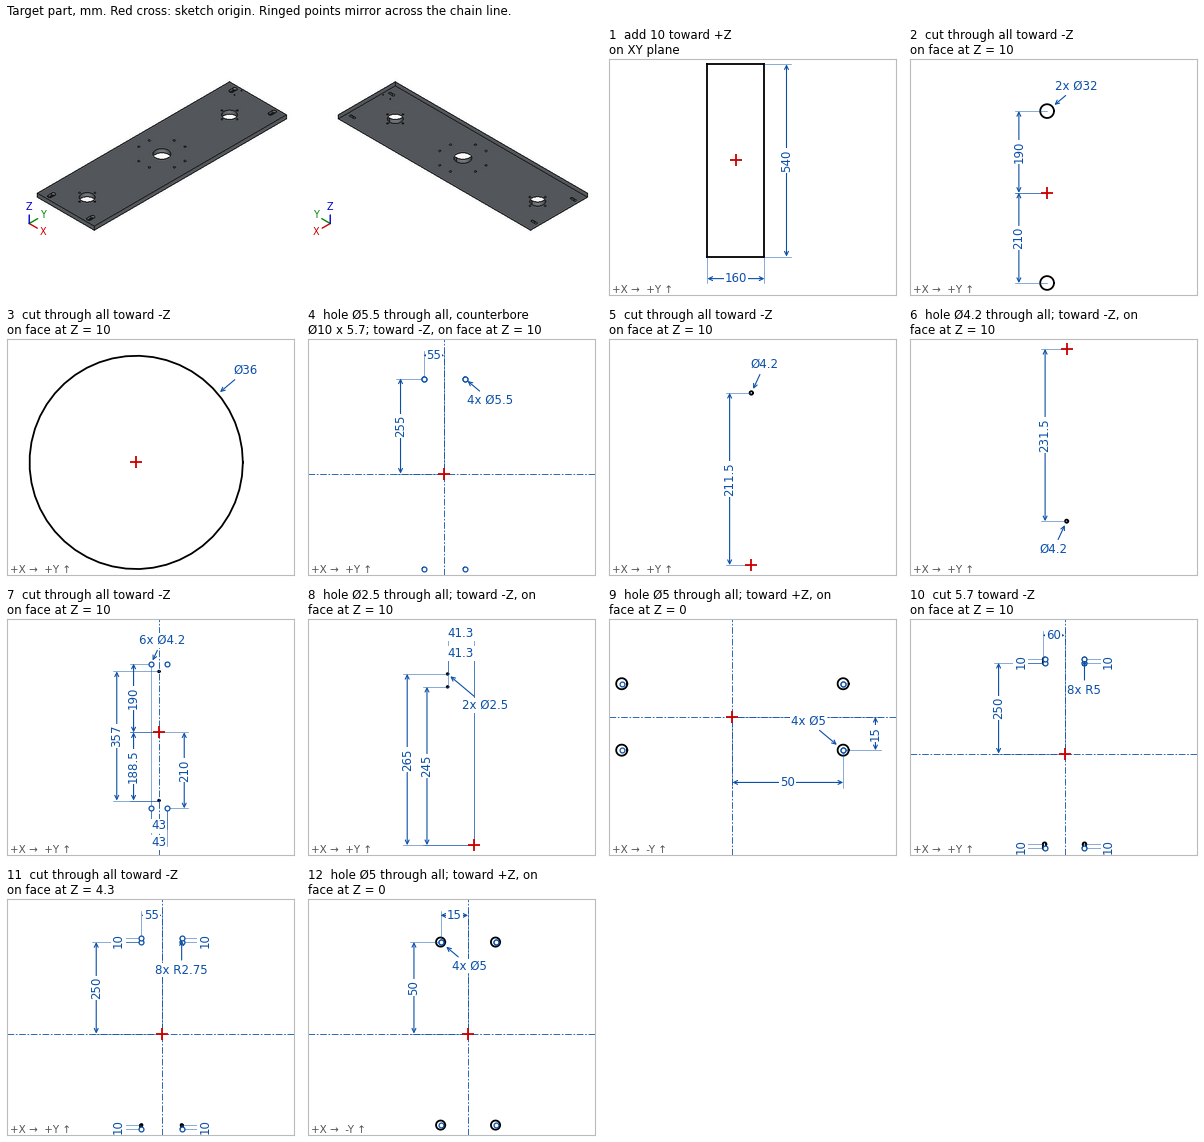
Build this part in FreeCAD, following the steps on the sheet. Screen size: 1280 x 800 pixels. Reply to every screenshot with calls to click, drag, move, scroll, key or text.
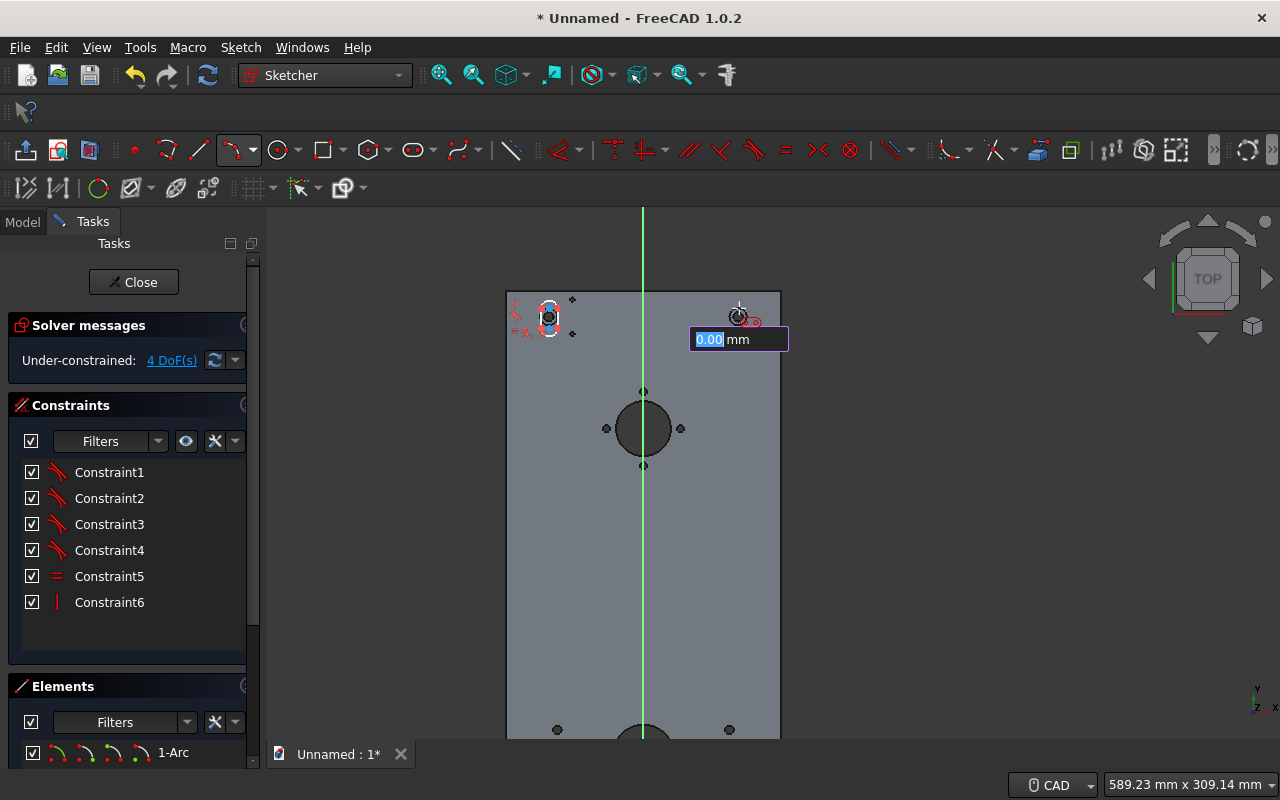
scroll(747, 317, up, 4)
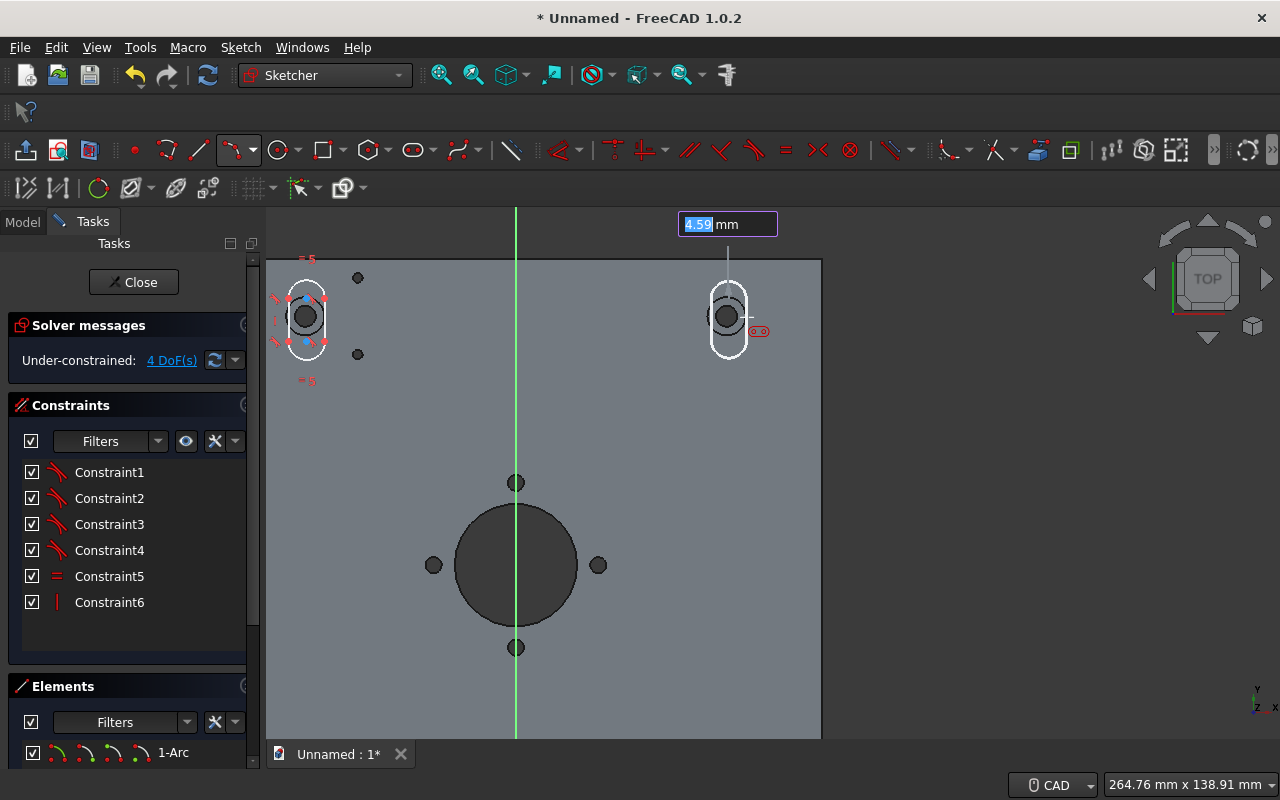
click(746, 316)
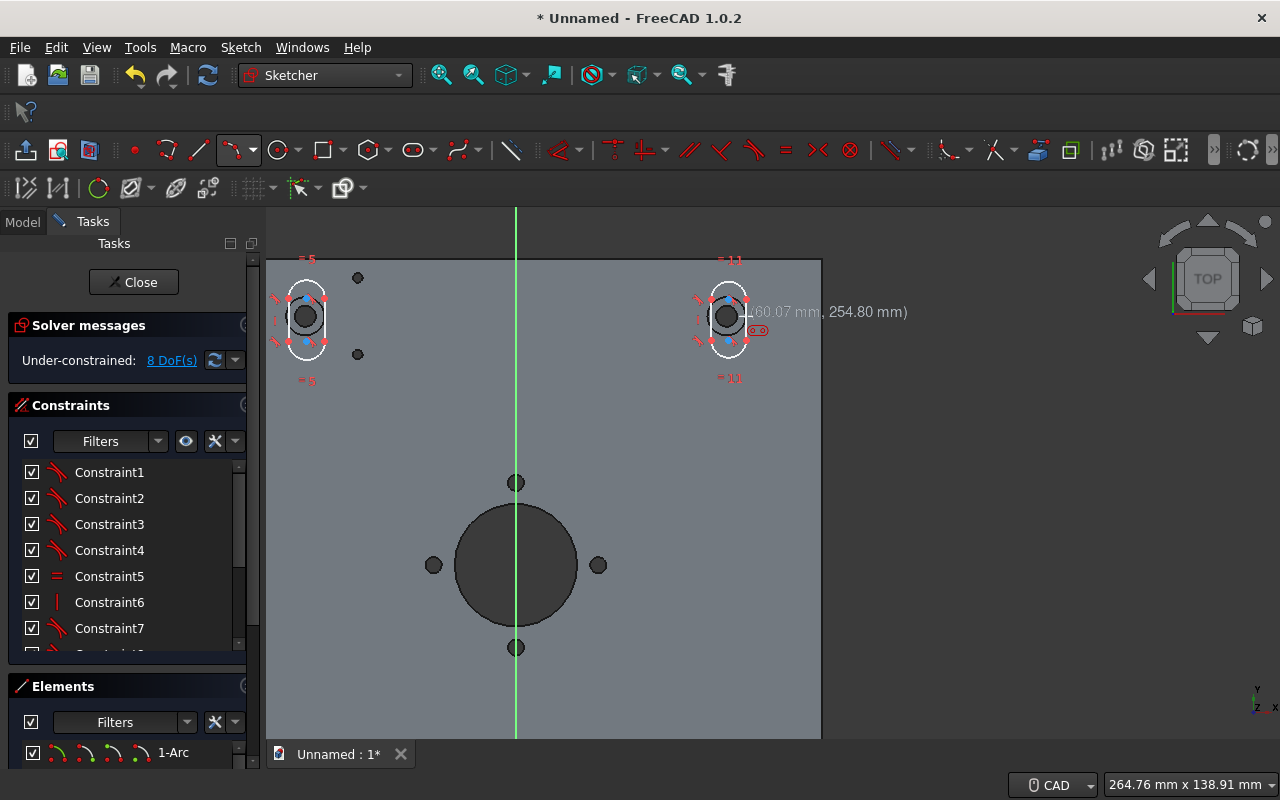
scroll(742, 311, down, 9)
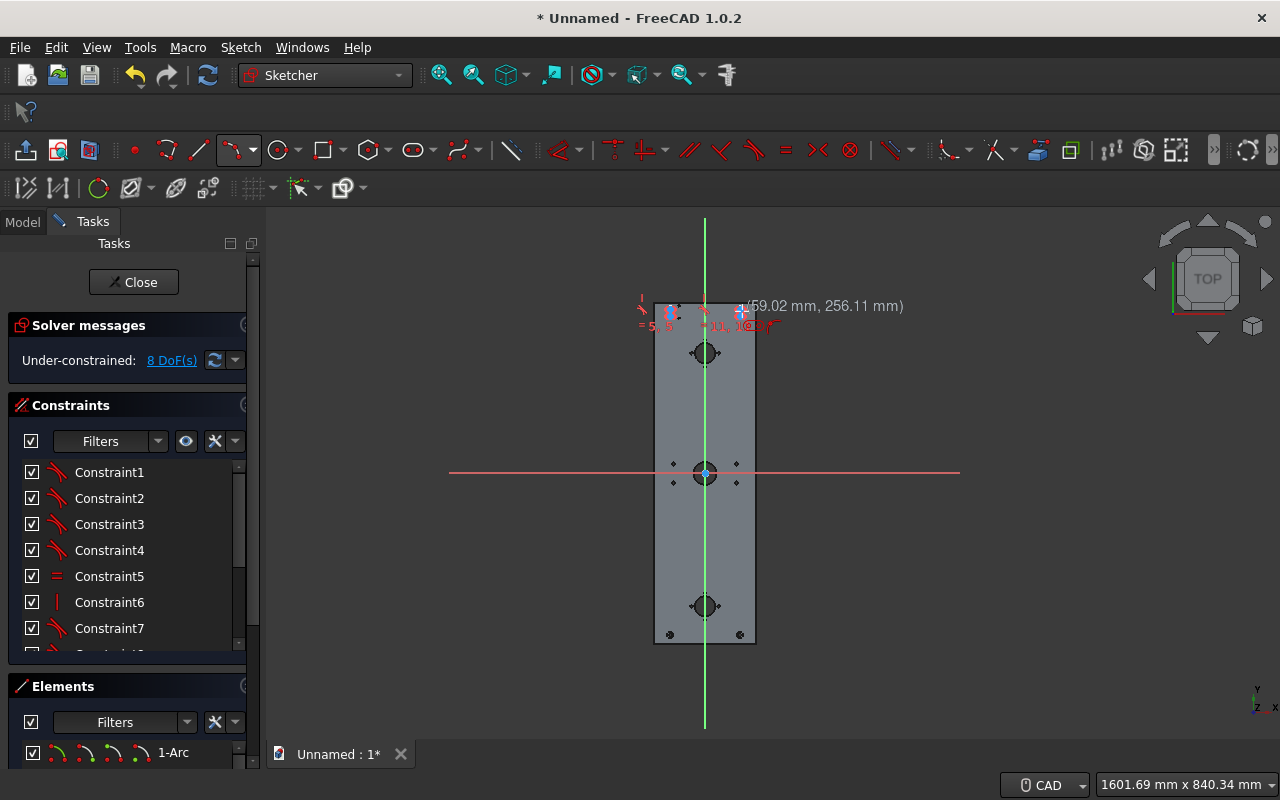
scroll(670, 638, up, 10)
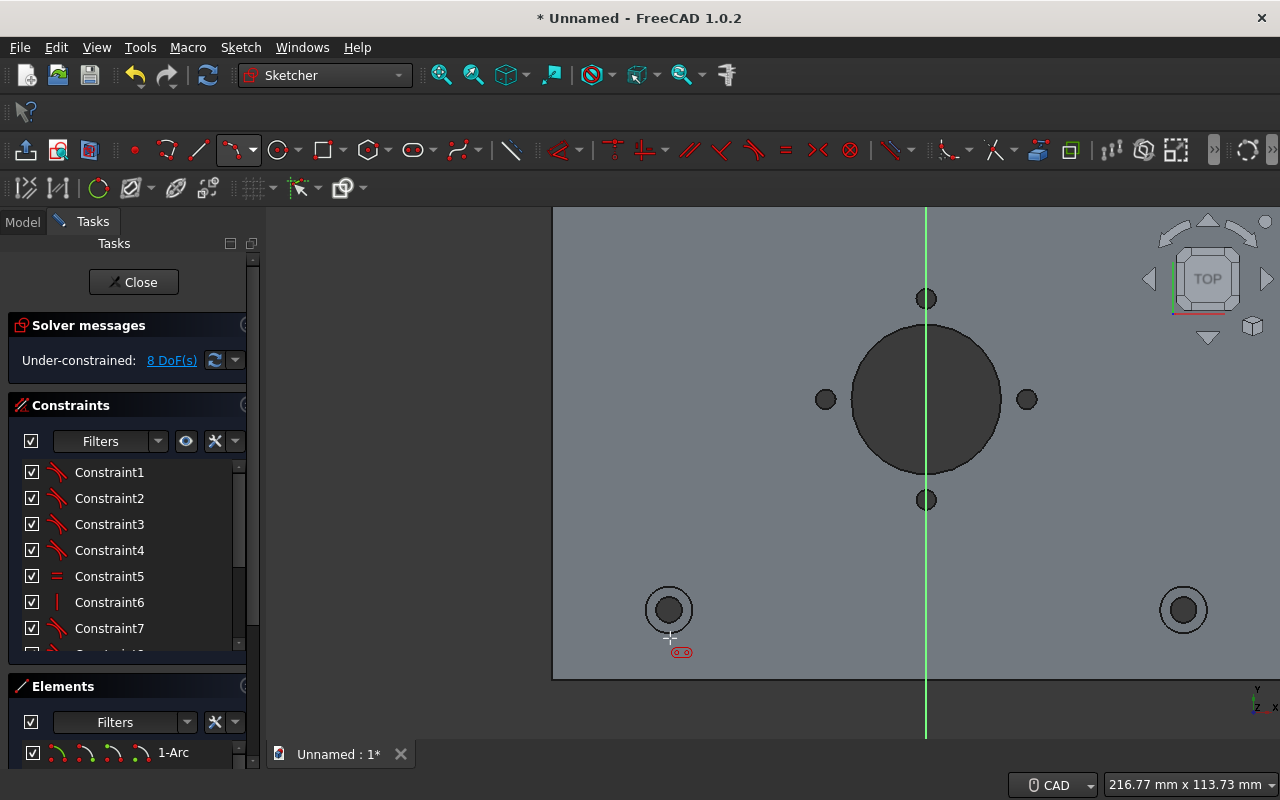
scroll(670, 638, down, 10)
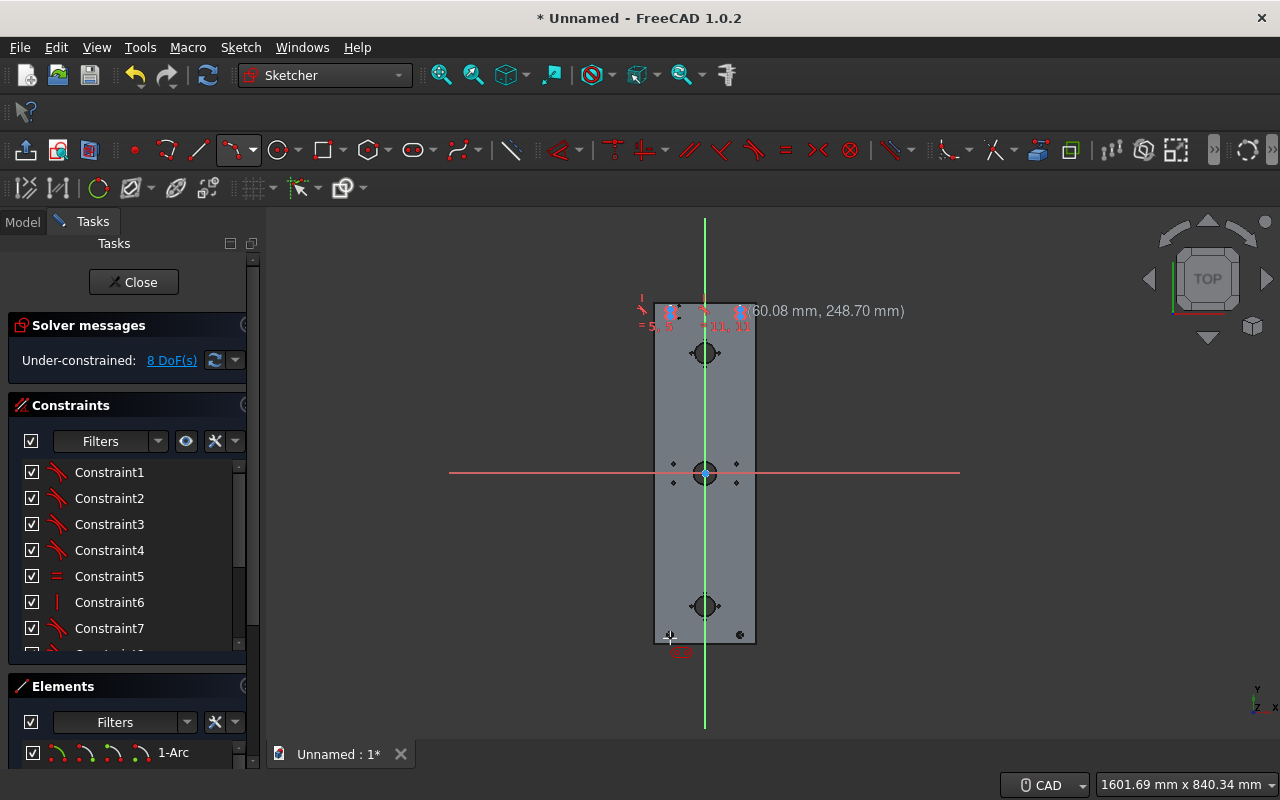
click(670, 638)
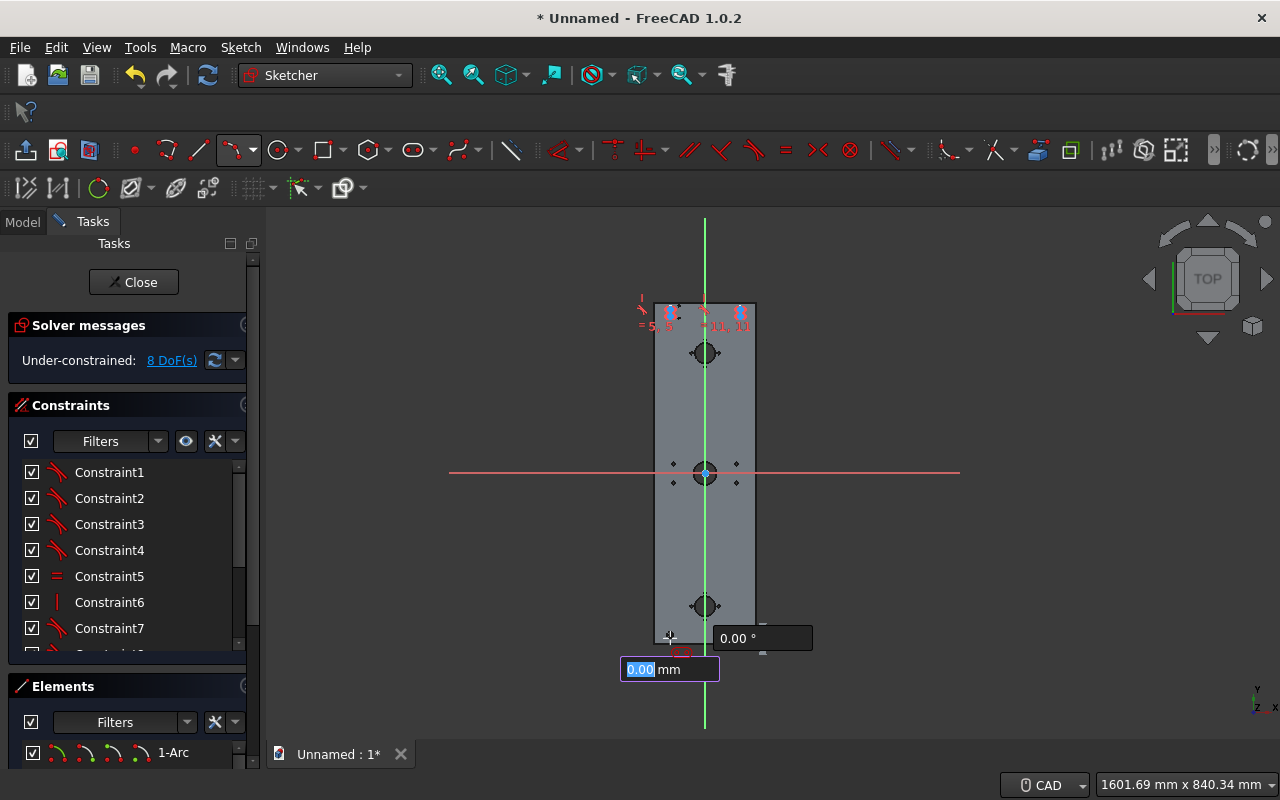
scroll(670, 632, up, 5)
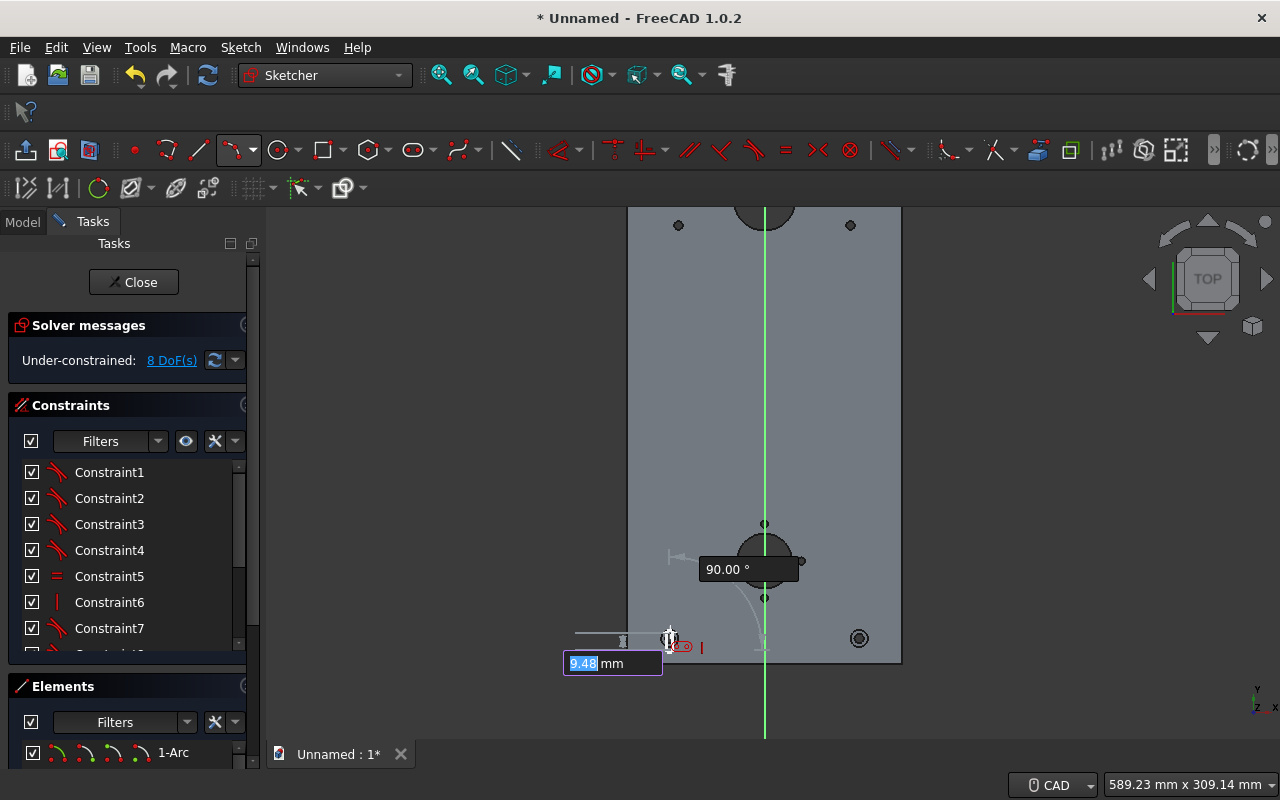
click(669, 630)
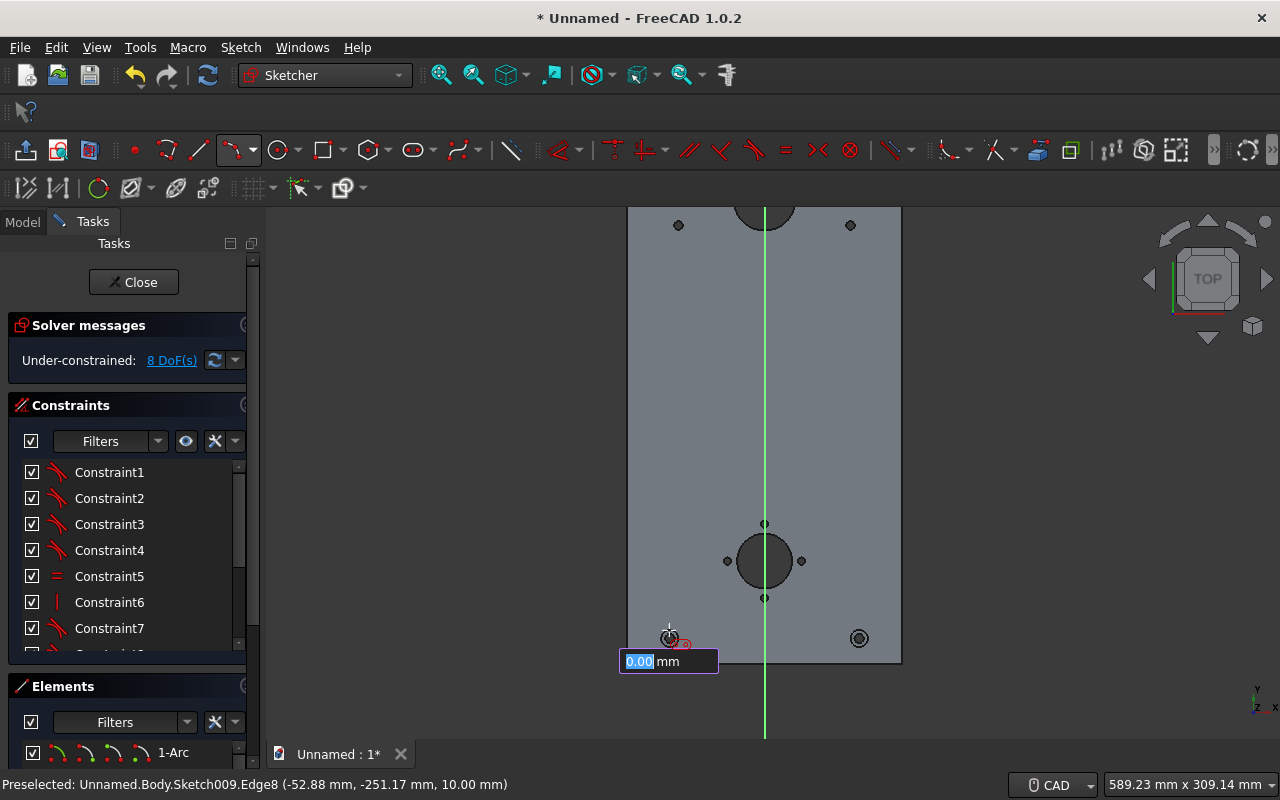
scroll(678, 639, up, 4)